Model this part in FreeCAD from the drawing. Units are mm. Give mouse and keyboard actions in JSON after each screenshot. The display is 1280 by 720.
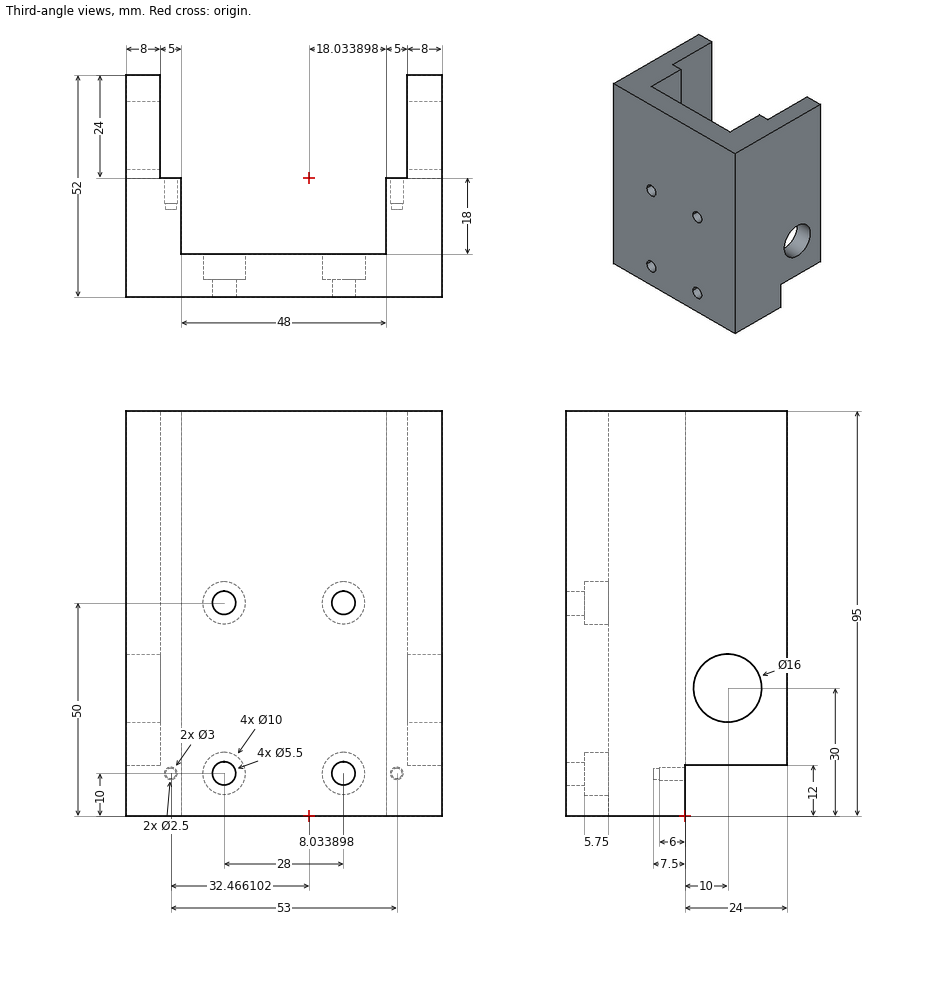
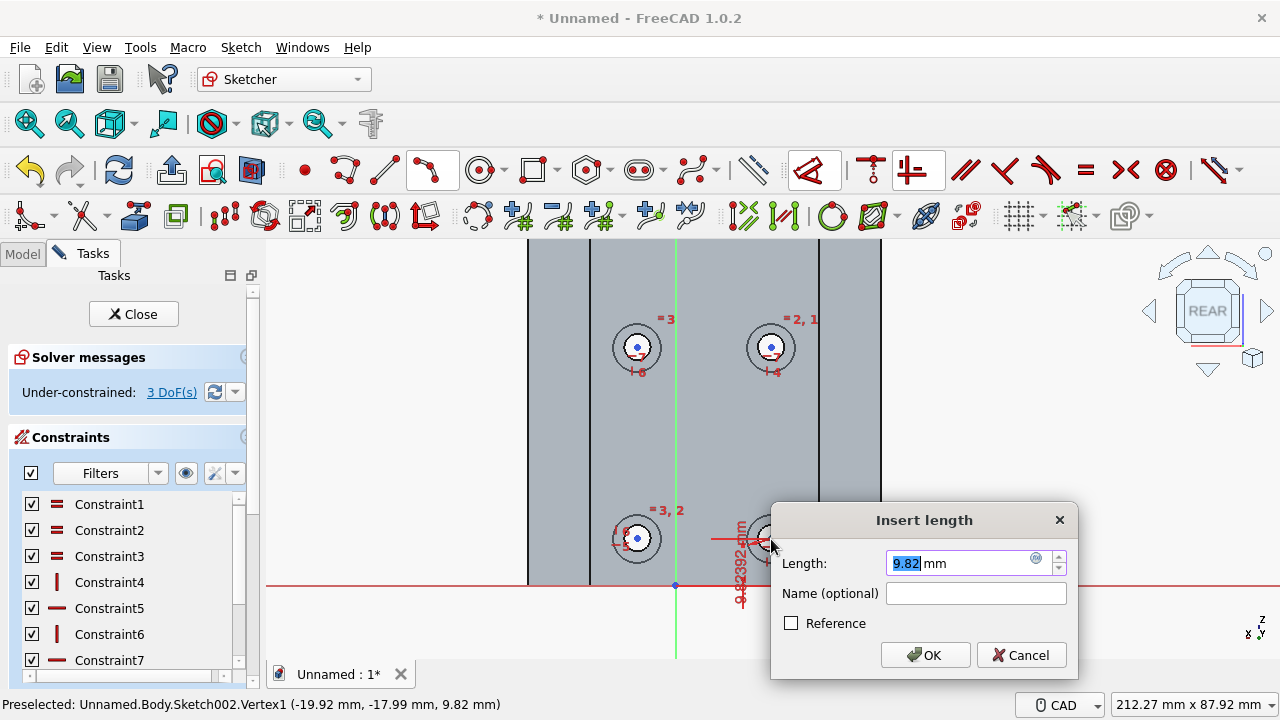
{"action": "type", "text": "10"}
{"action": "key", "text": "Return"}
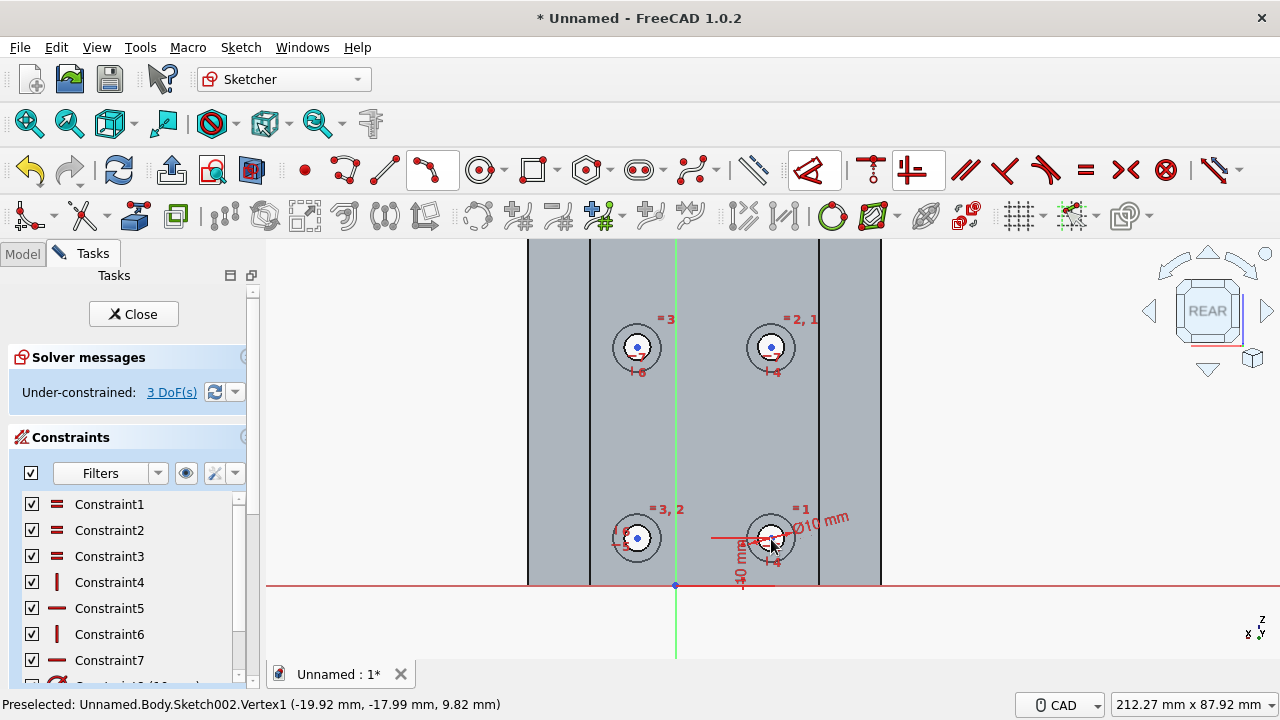
{"action": "left_click", "coordinate": [771, 348]}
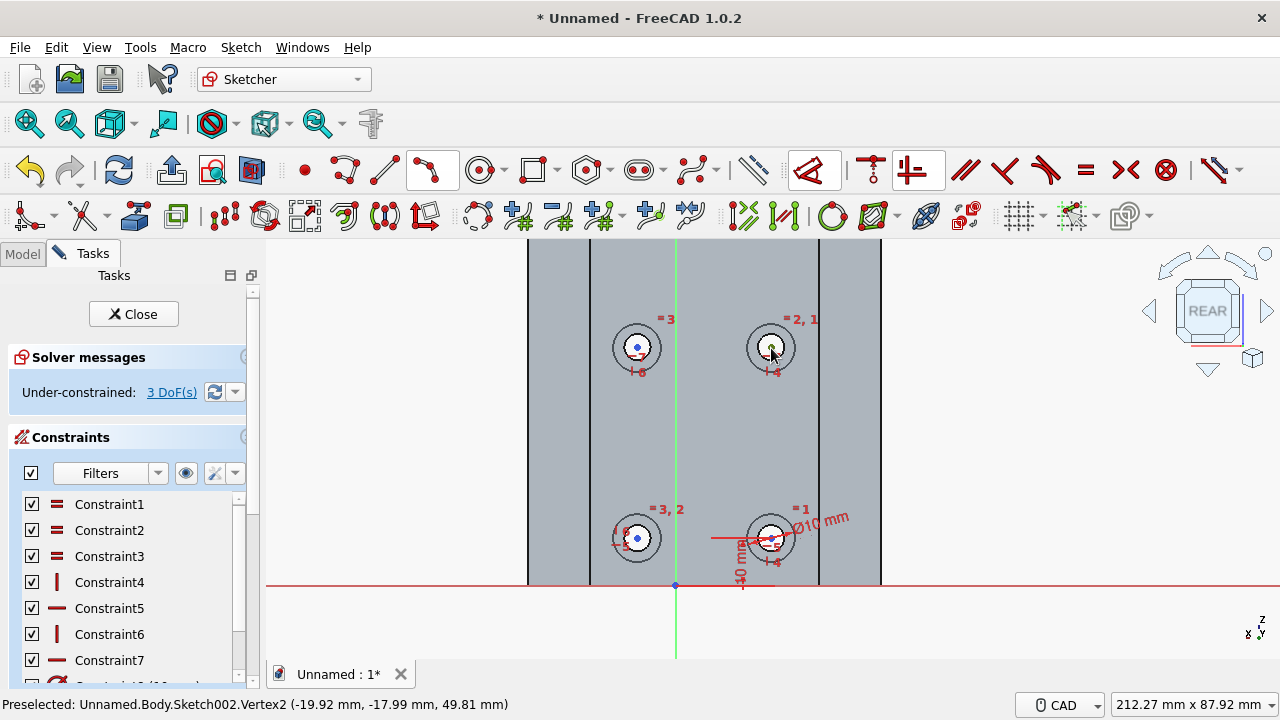
{"action": "left_click", "coordinate": [836, 170]}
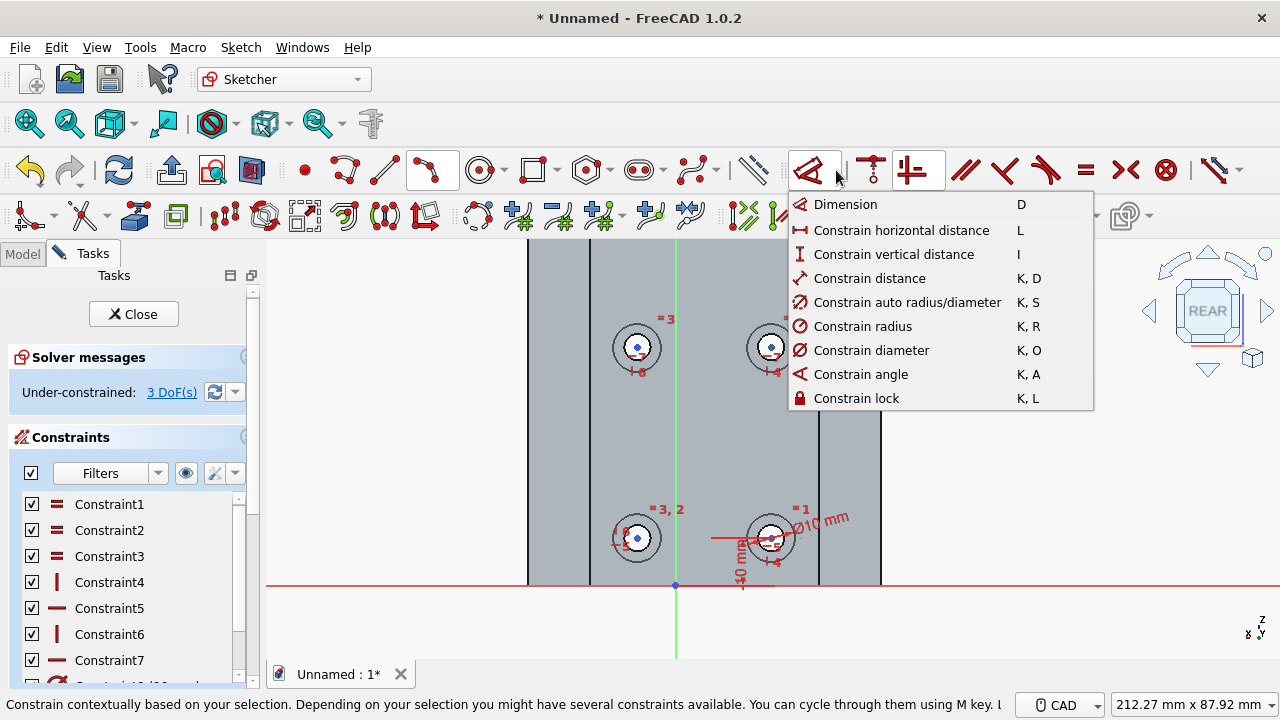
{"action": "left_click", "coordinate": [941, 254]}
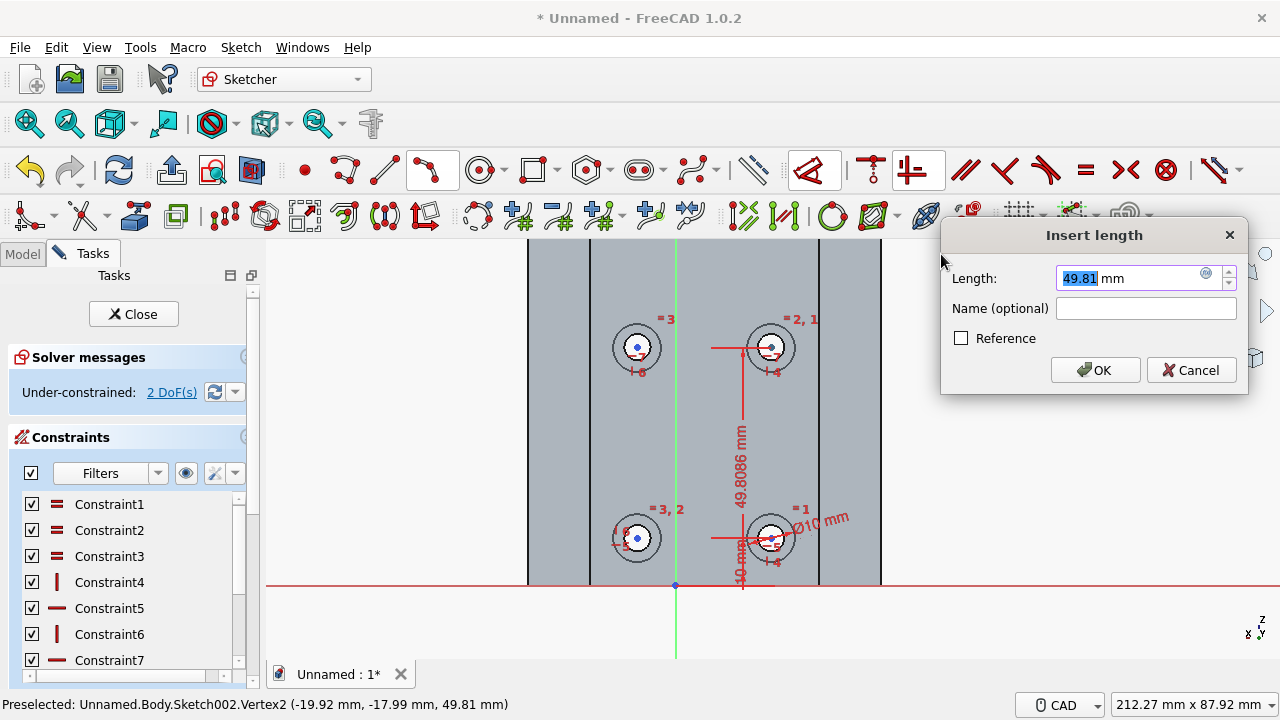
{"action": "type", "text": "50"}
{"action": "key", "text": "Return"}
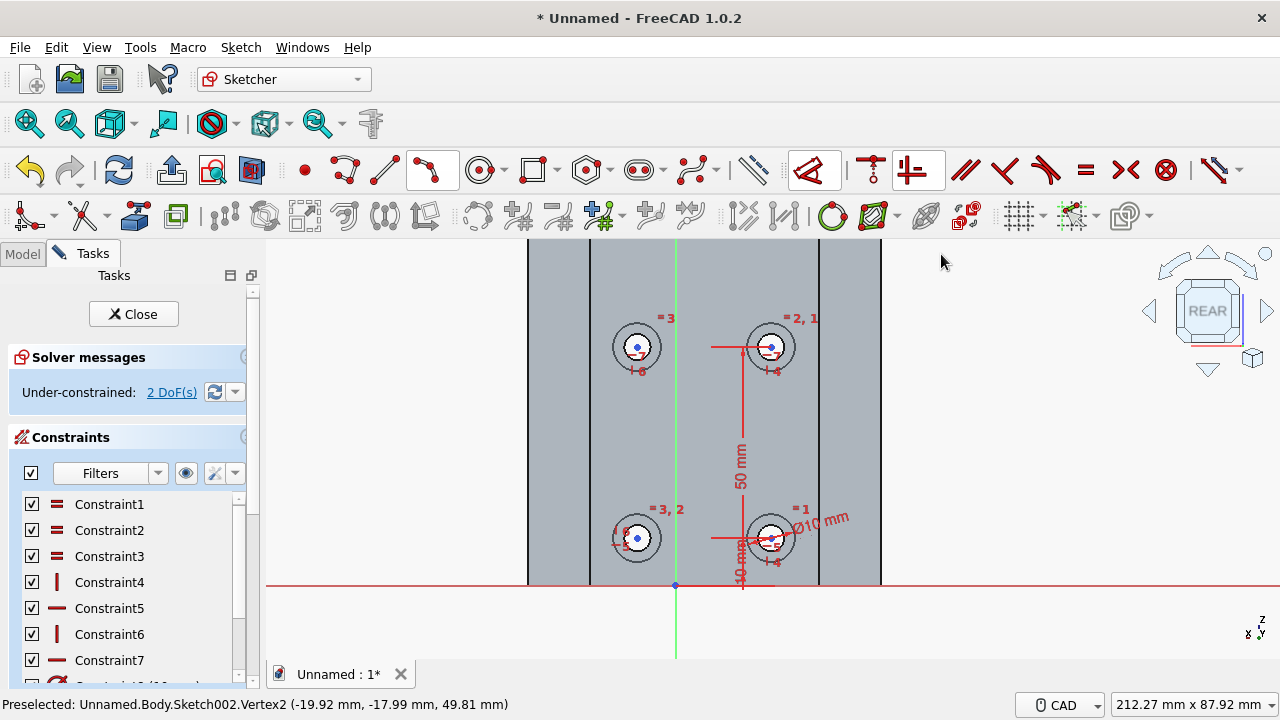
{"action": "left_click", "coordinate": [771, 538]}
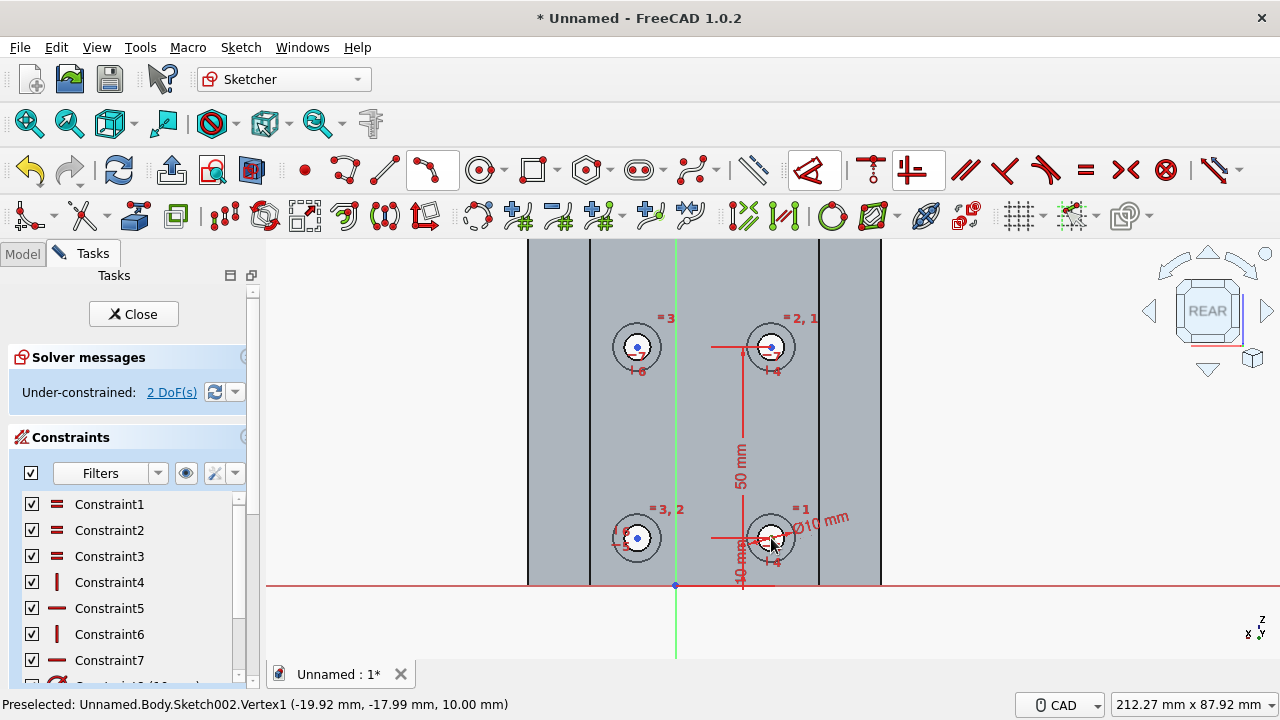
{"action": "left_click", "coordinate": [637, 538]}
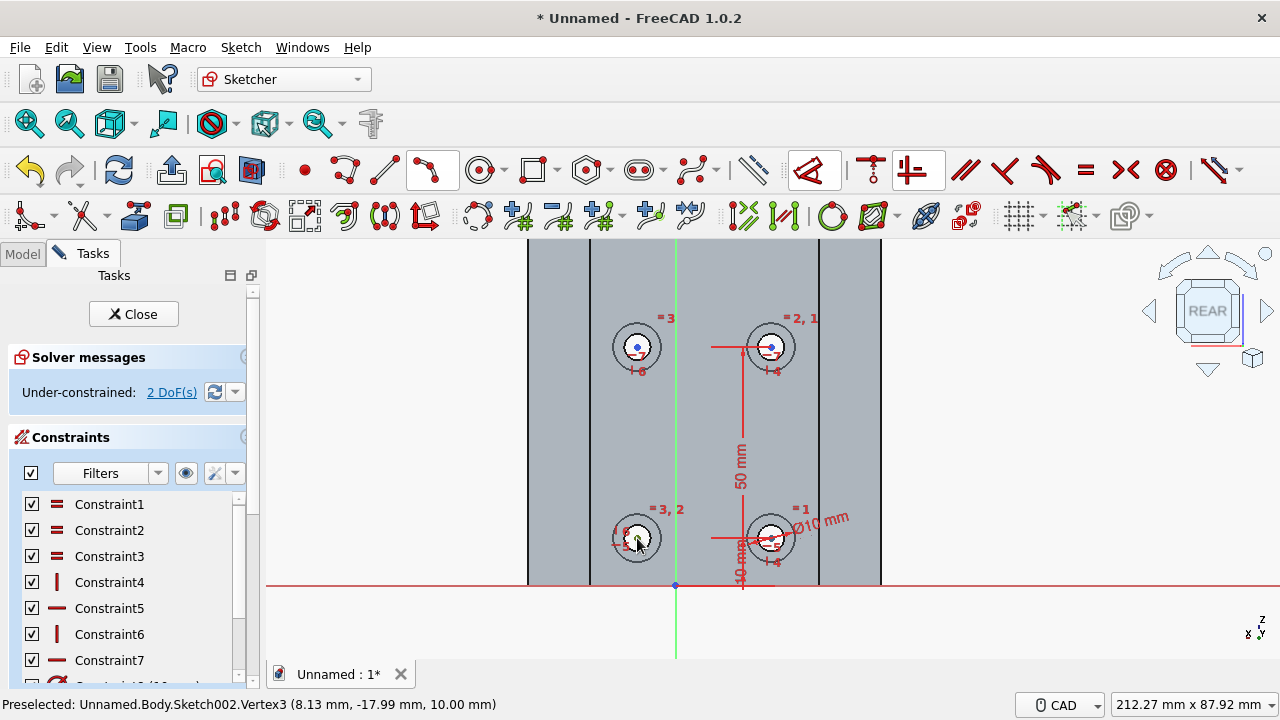
{"action": "key", "text": "l"}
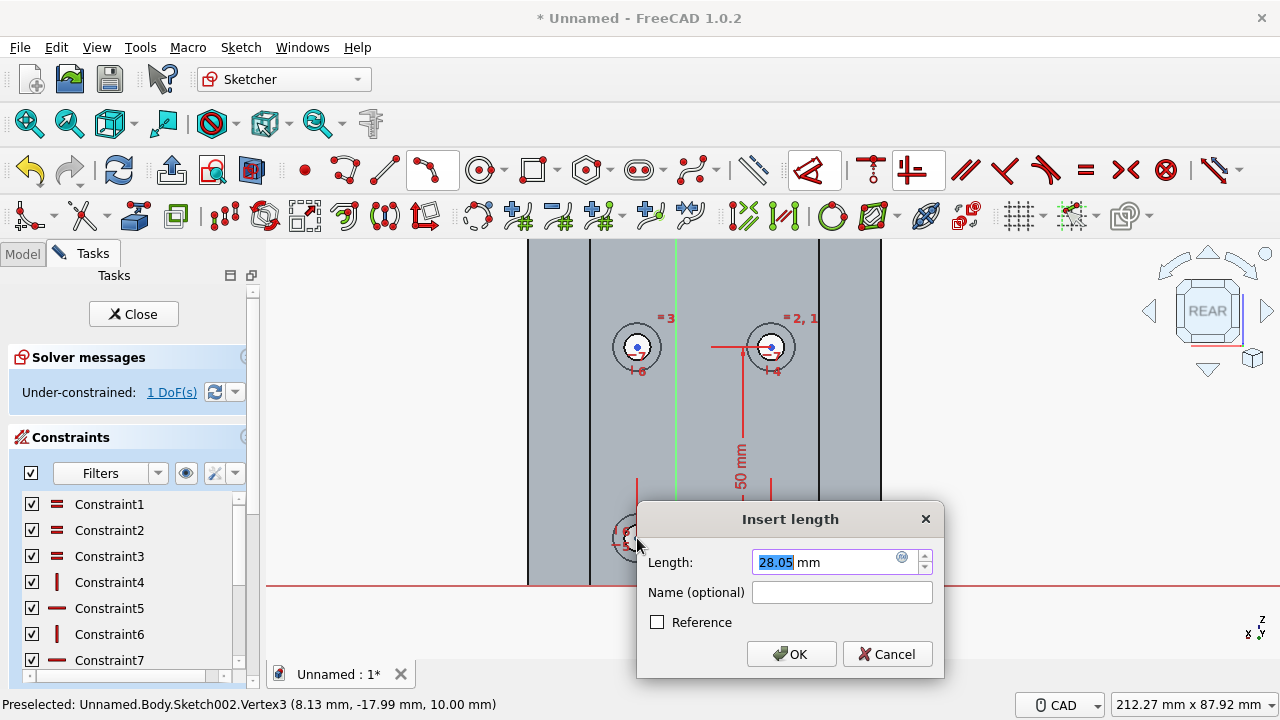
{"action": "type", "text": "28"}
{"action": "key", "text": "Return"}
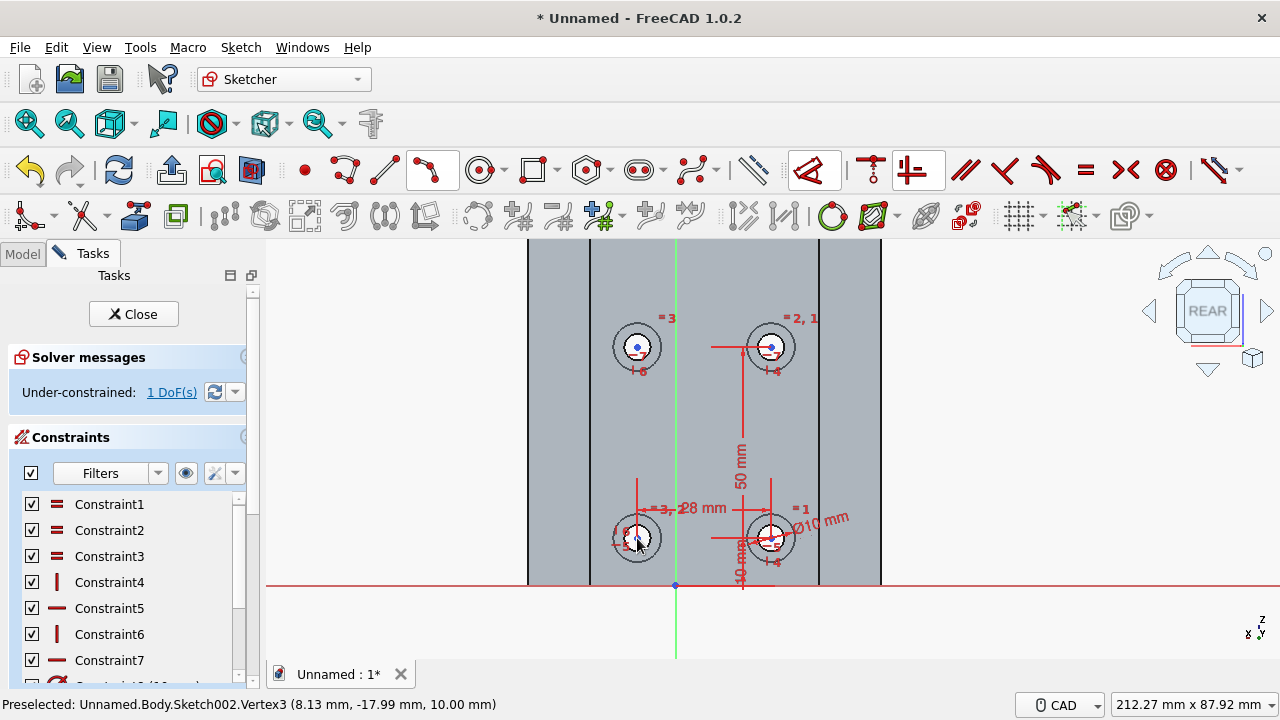
{"action": "left_click", "coordinate": [637, 538]}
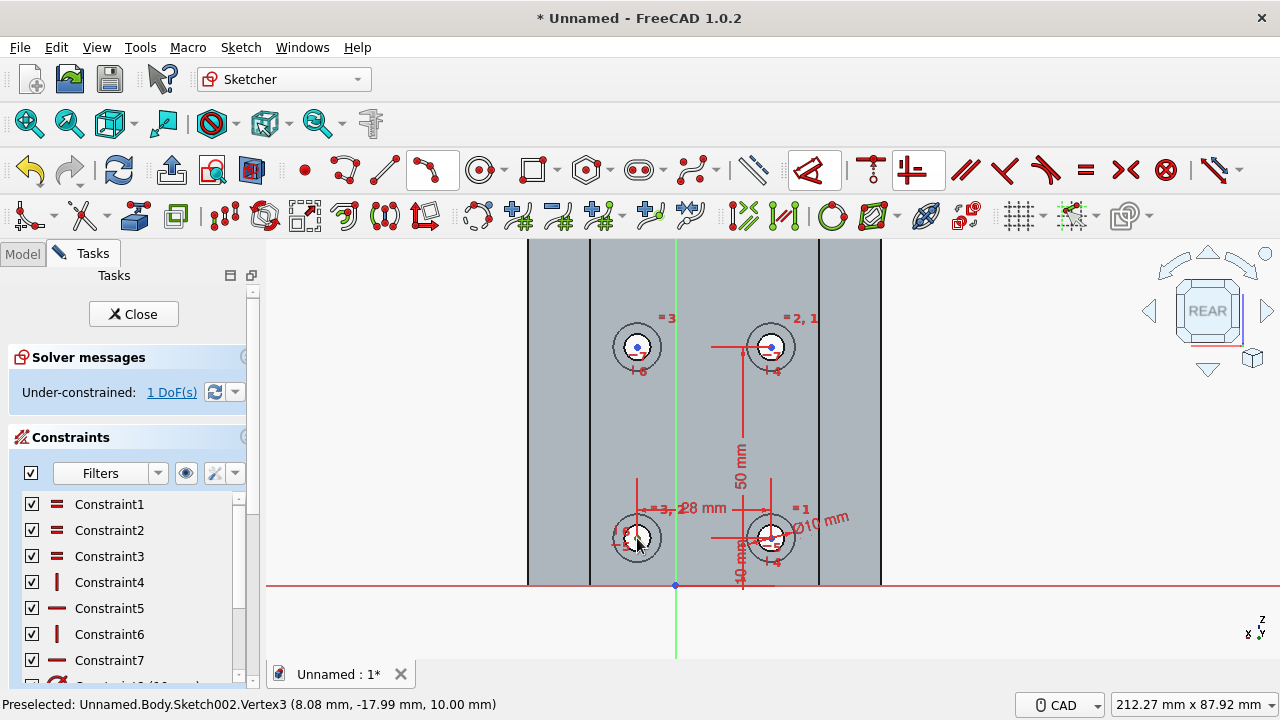
{"action": "key", "text": "l"}